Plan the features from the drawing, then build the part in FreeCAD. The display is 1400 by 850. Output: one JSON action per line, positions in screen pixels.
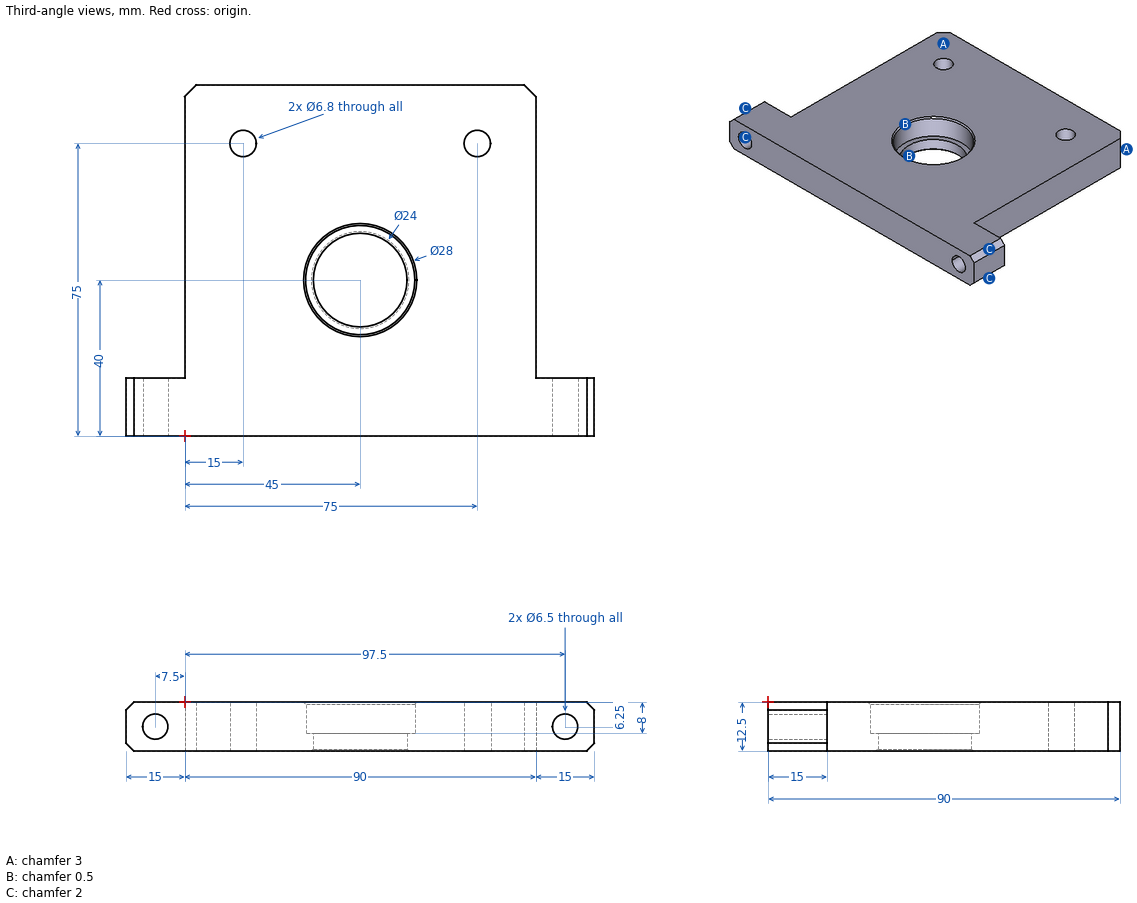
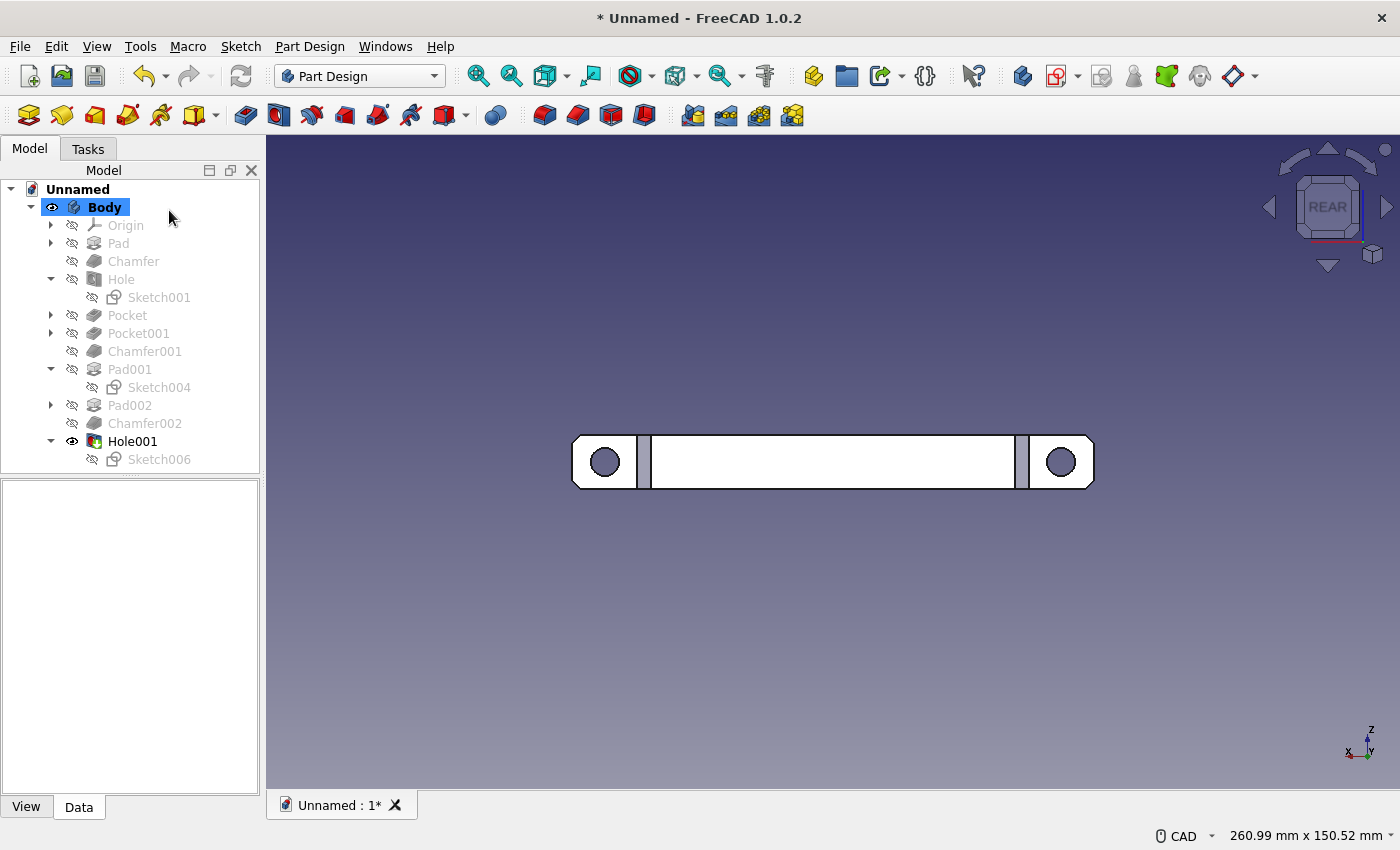
{"action": "key", "text": "0"}